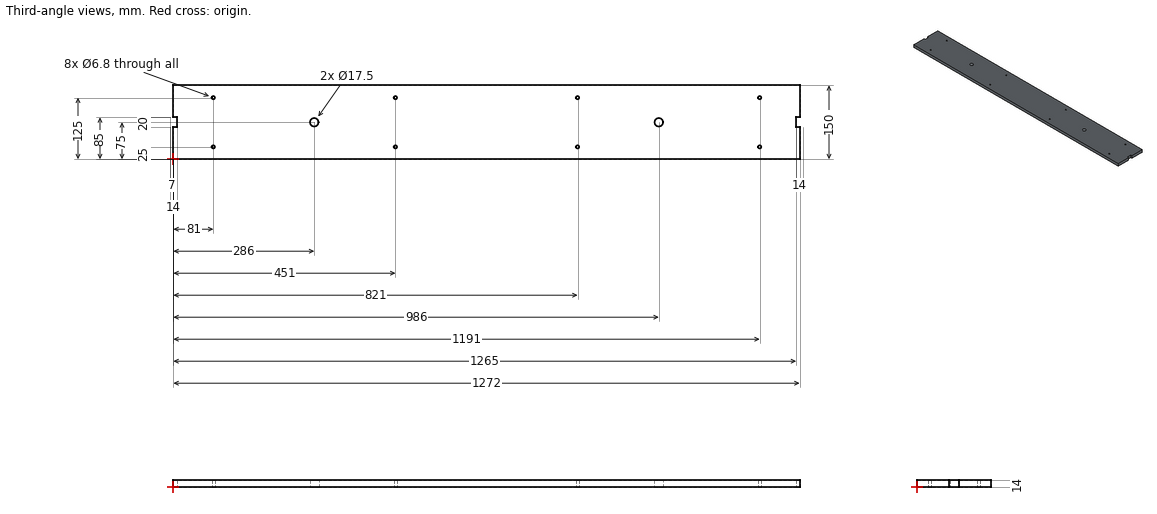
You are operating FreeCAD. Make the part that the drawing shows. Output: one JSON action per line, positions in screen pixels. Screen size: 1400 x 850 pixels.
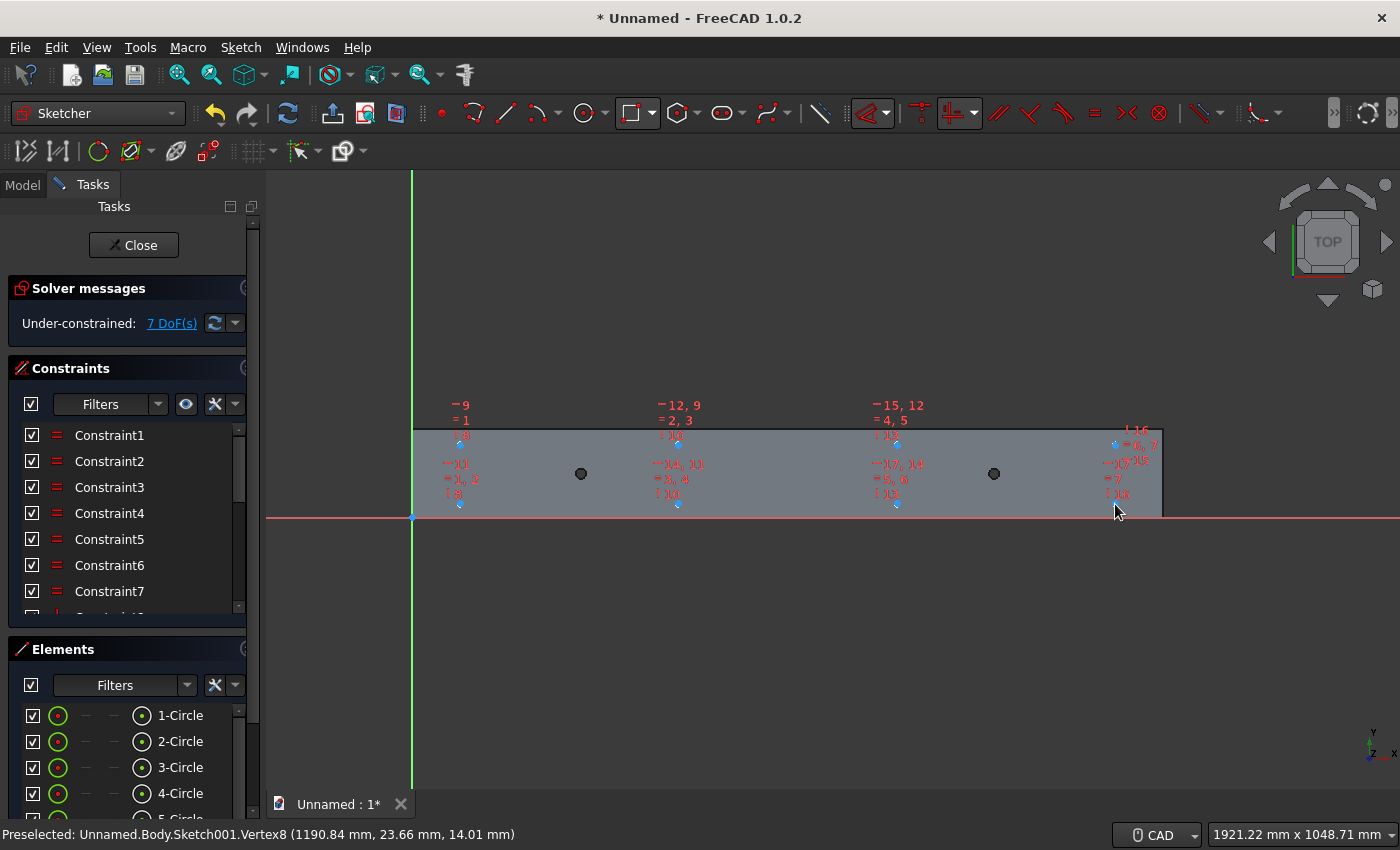
{"action": "scroll", "coordinate": [458, 445], "scroll_direction": "up", "scroll_amount": 12}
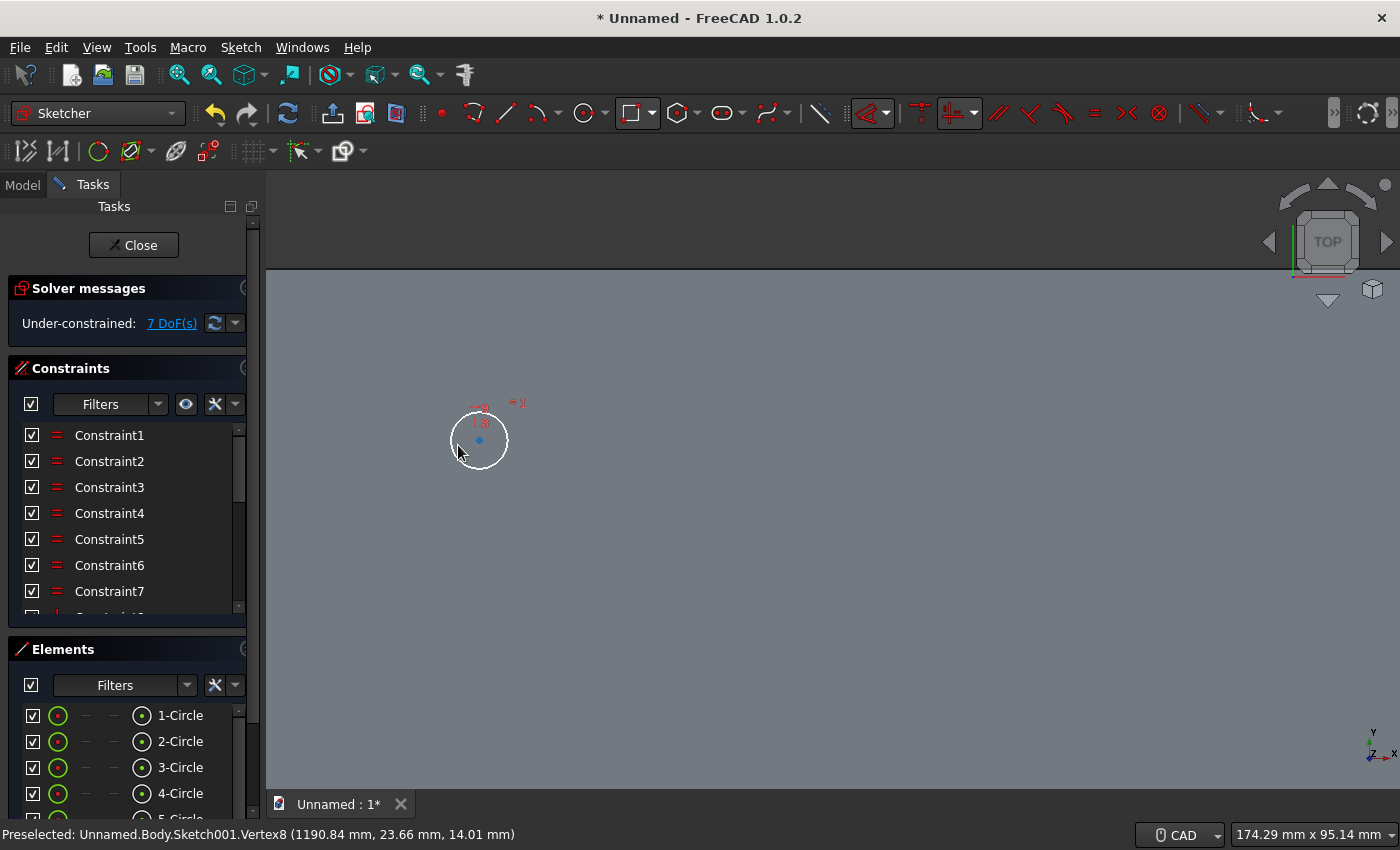
{"action": "left_click", "coordinate": [451, 440]}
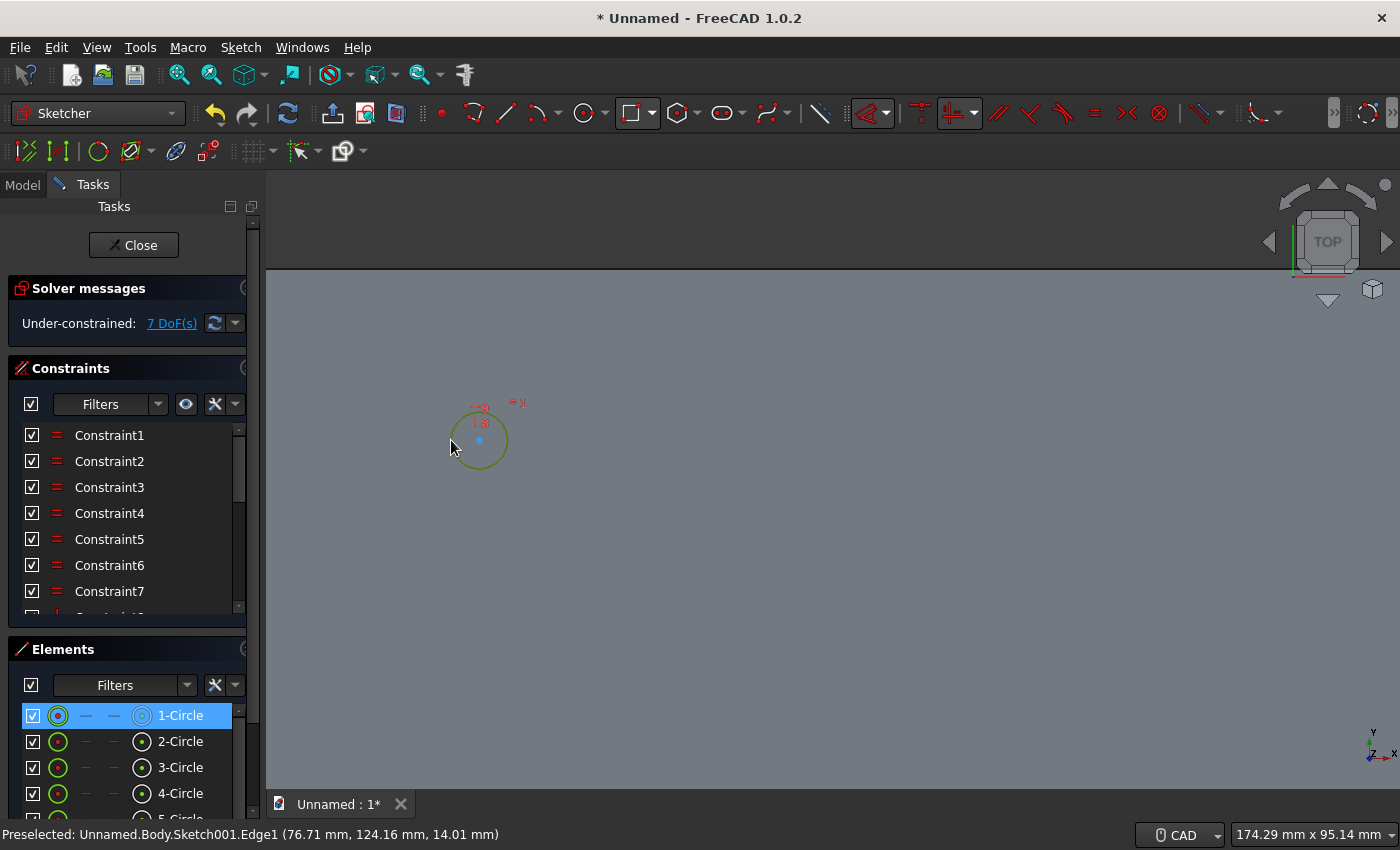
{"action": "key", "text": "k o"}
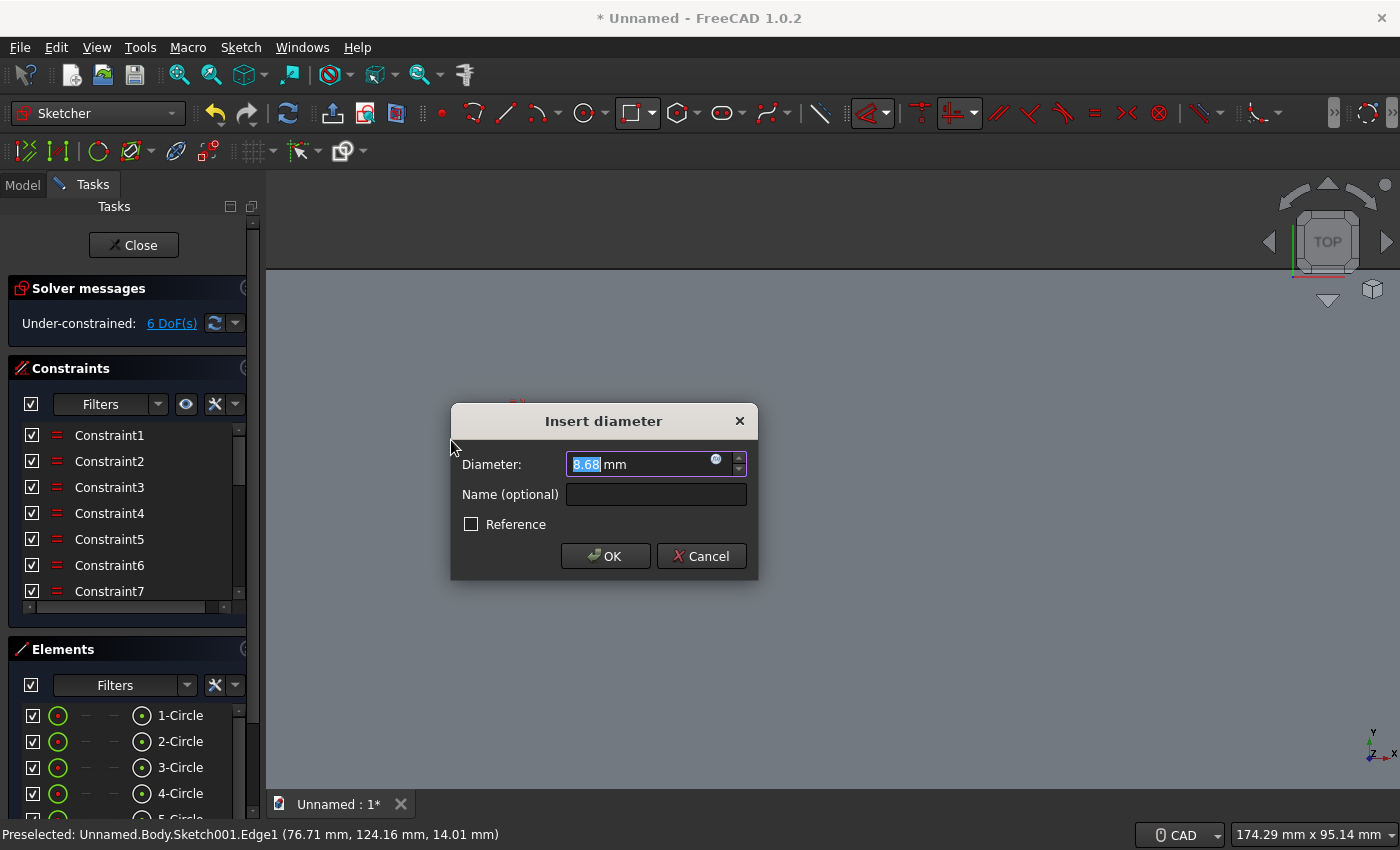
{"action": "type", "text": "6.8"}
{"action": "key", "text": "Return"}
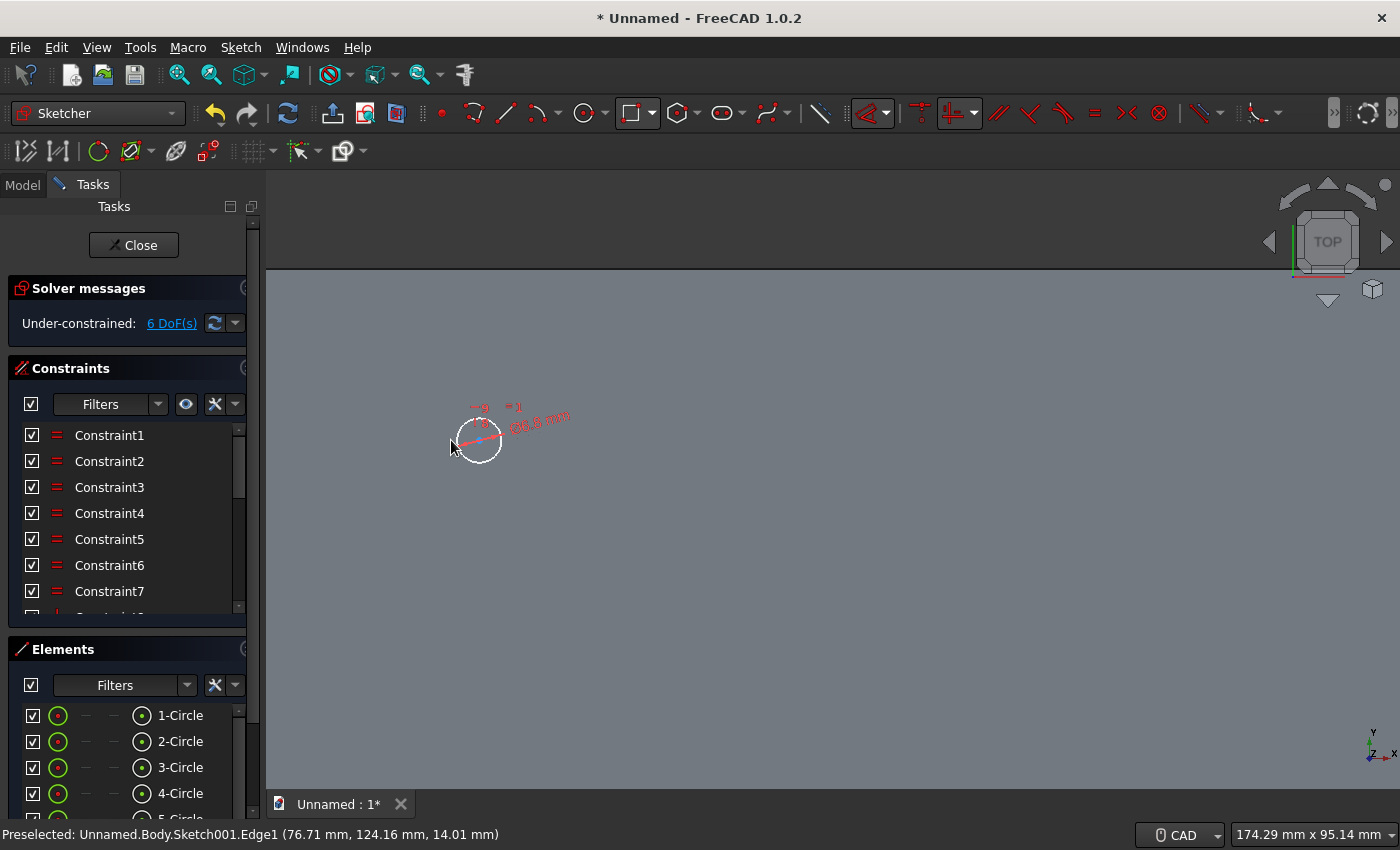
{"action": "scroll", "coordinate": [458, 445], "scroll_direction": "down", "scroll_amount": 12}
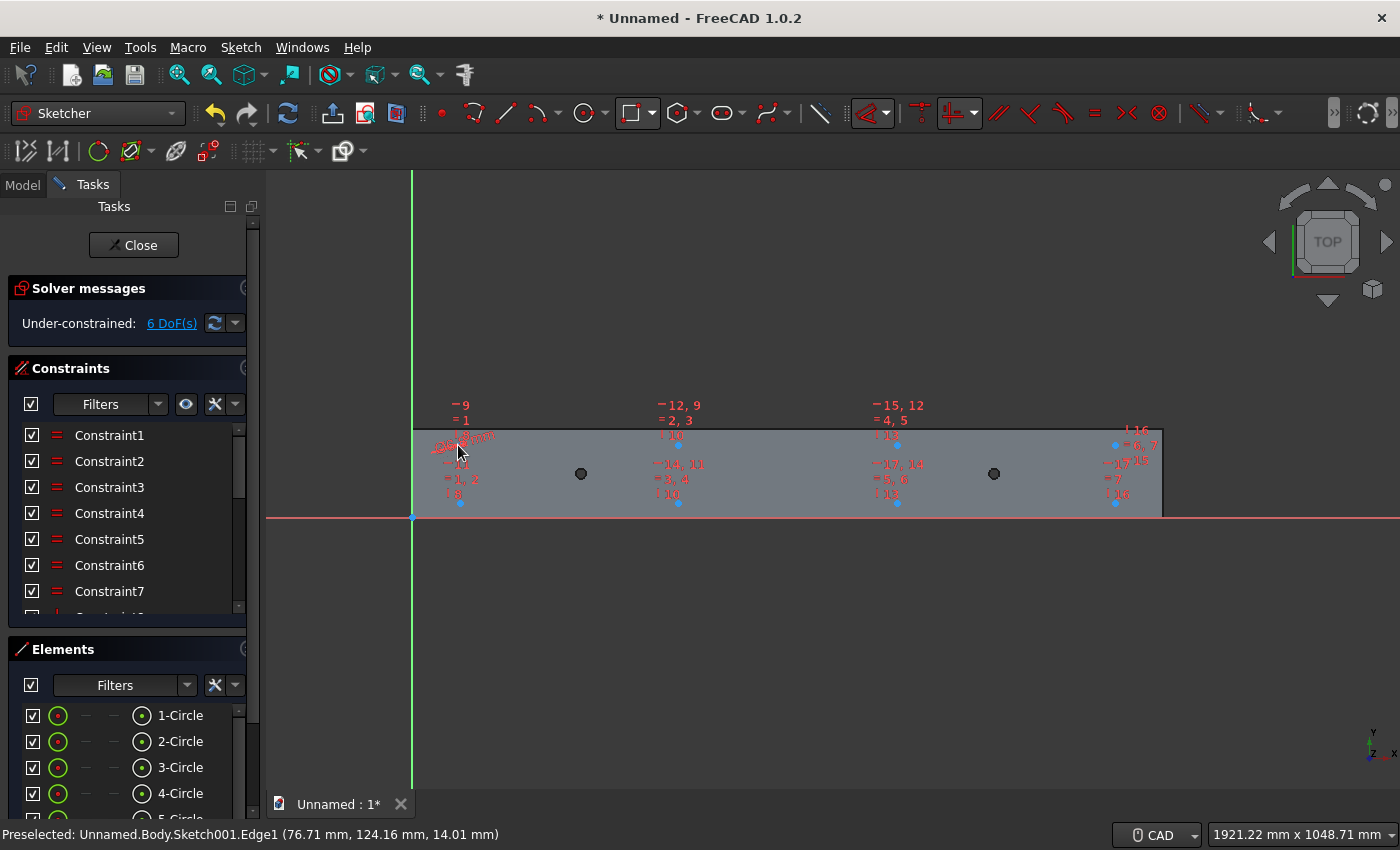
{"action": "left_click", "coordinate": [460, 445]}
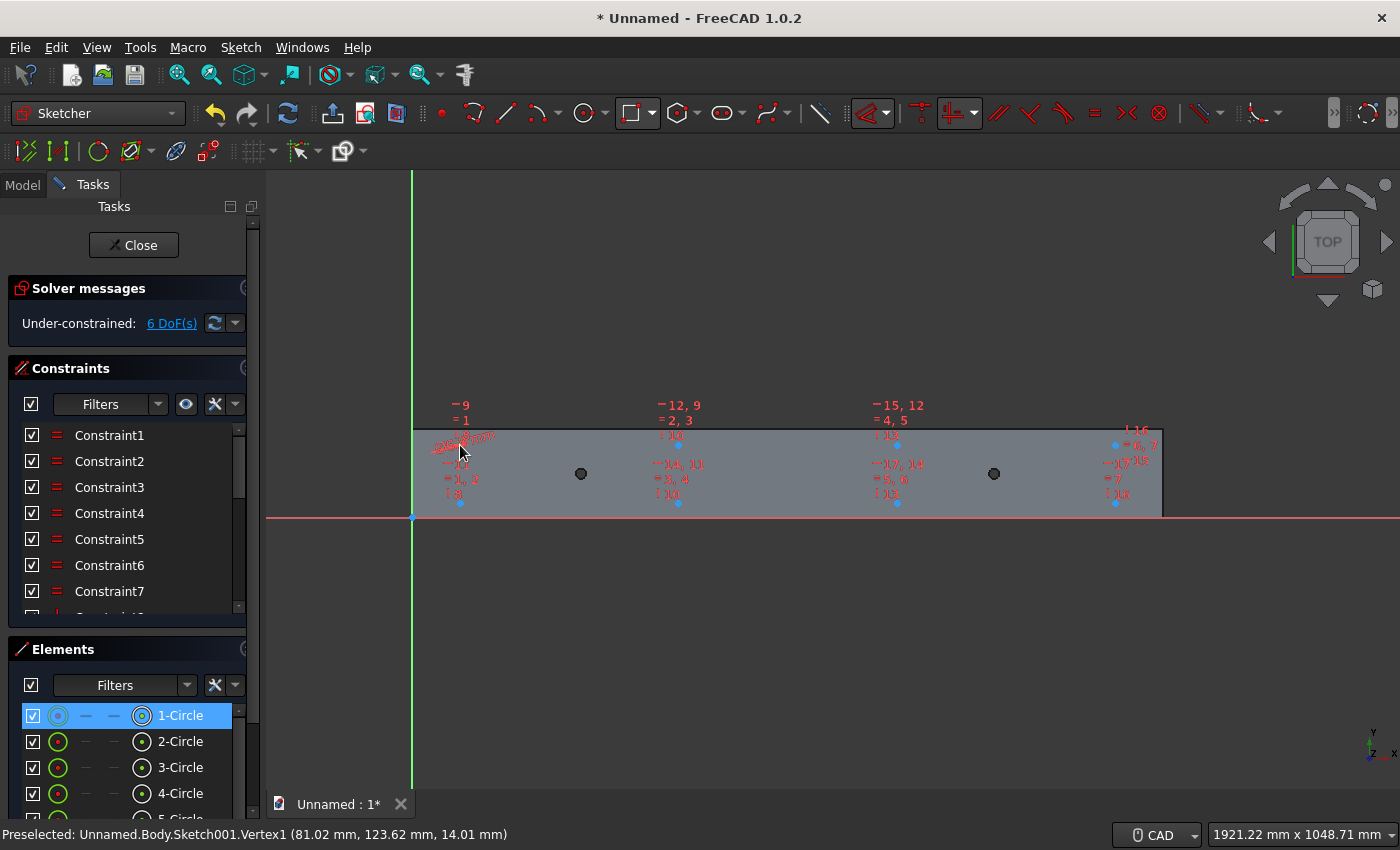
{"action": "key", "text": "l"}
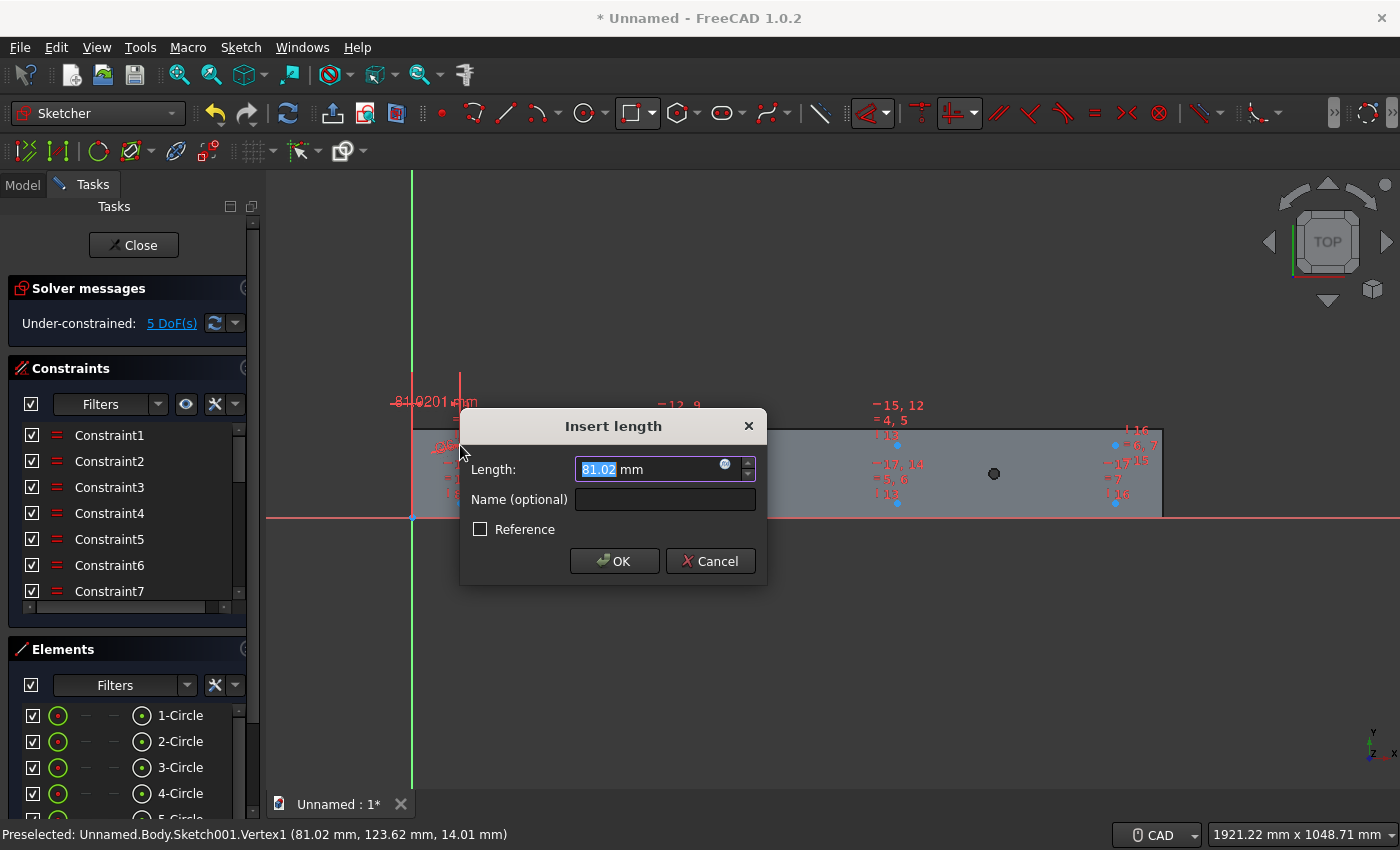
{"action": "type", "text": "81"}
{"action": "key", "text": "Return"}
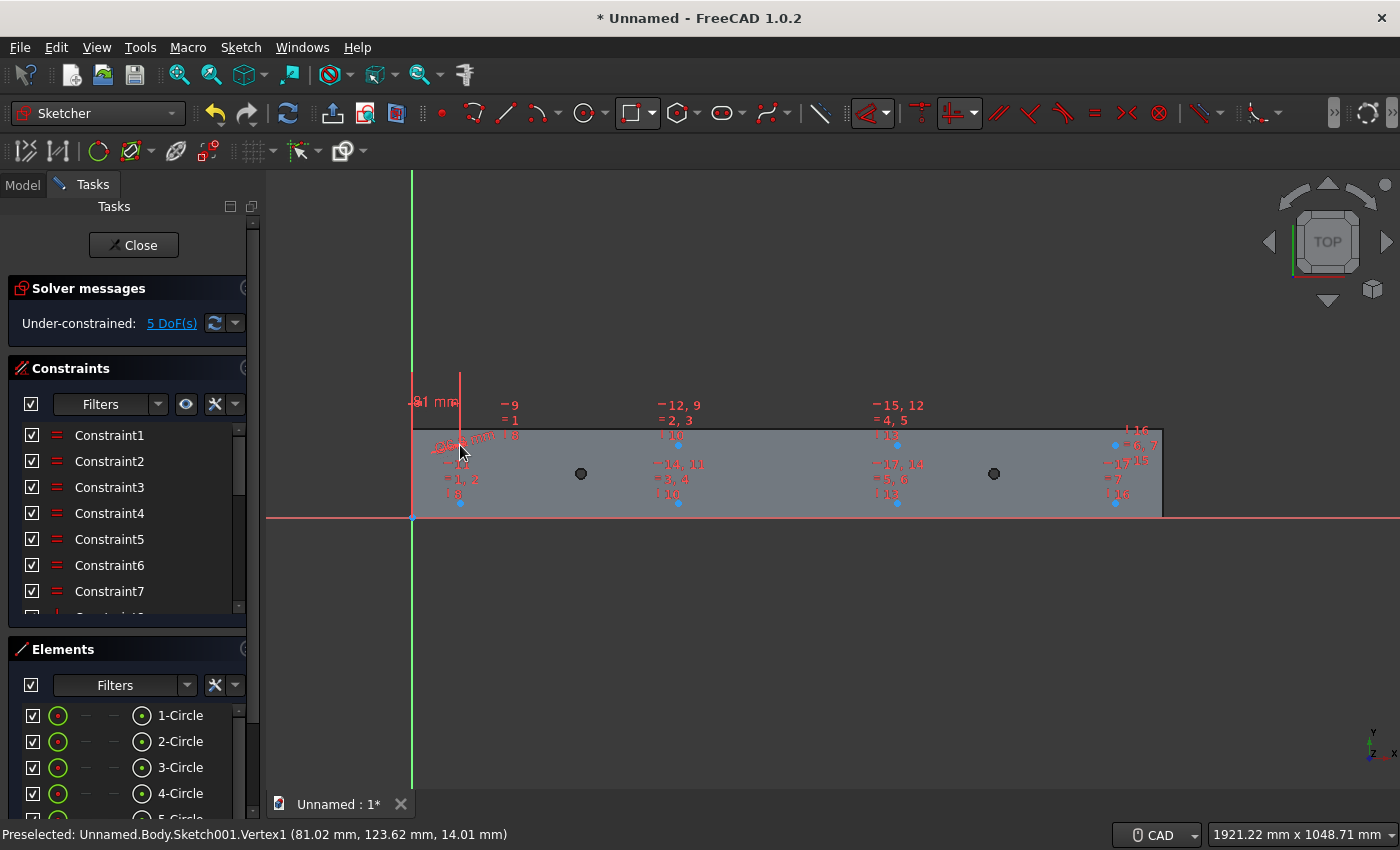
{"action": "scroll", "coordinate": [460, 504], "scroll_direction": "up", "scroll_amount": 5}